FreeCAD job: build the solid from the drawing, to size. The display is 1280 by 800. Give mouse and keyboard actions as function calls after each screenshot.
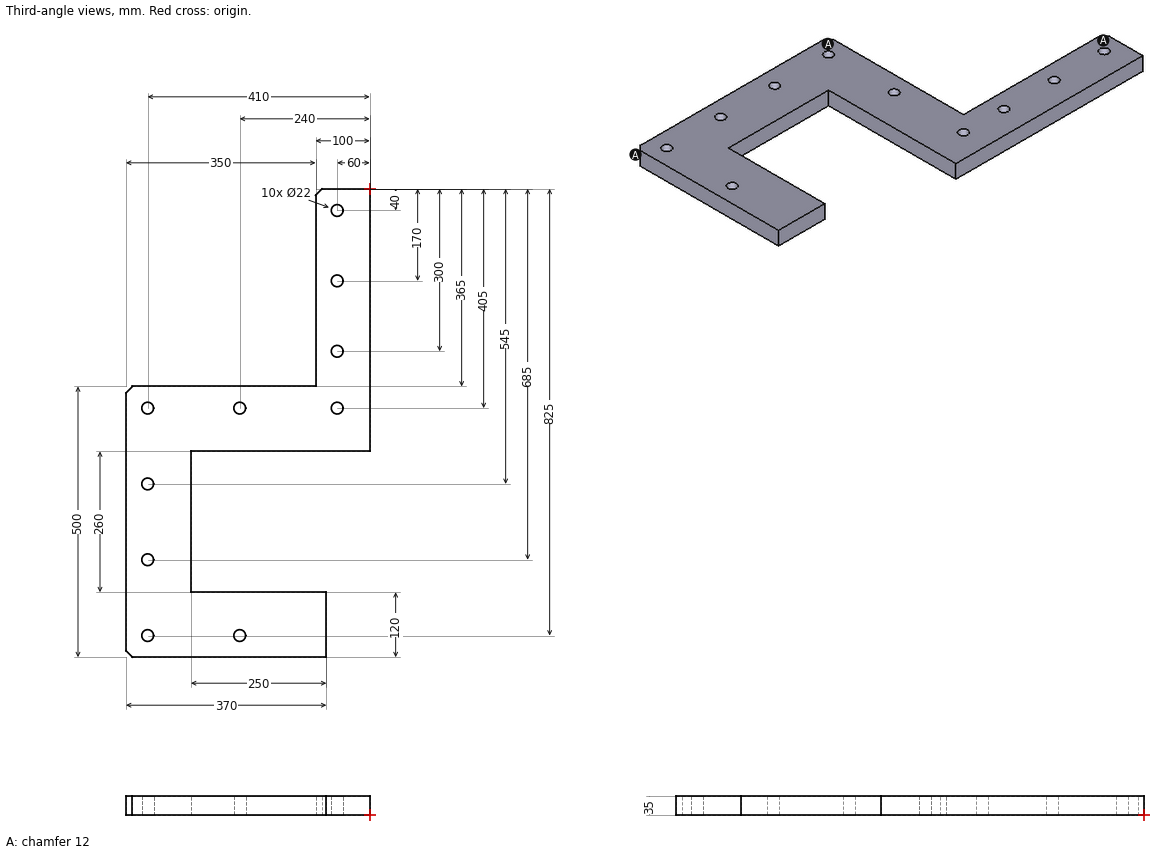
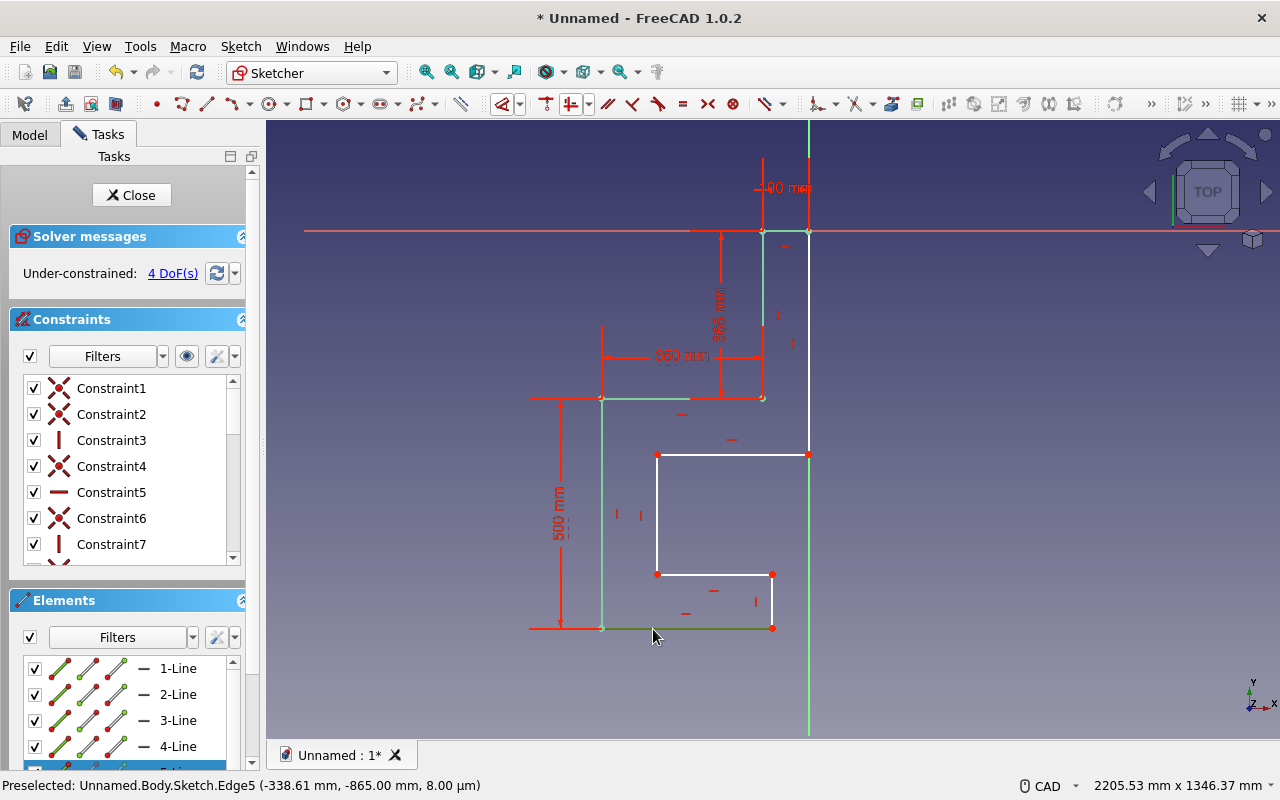
click(520, 104)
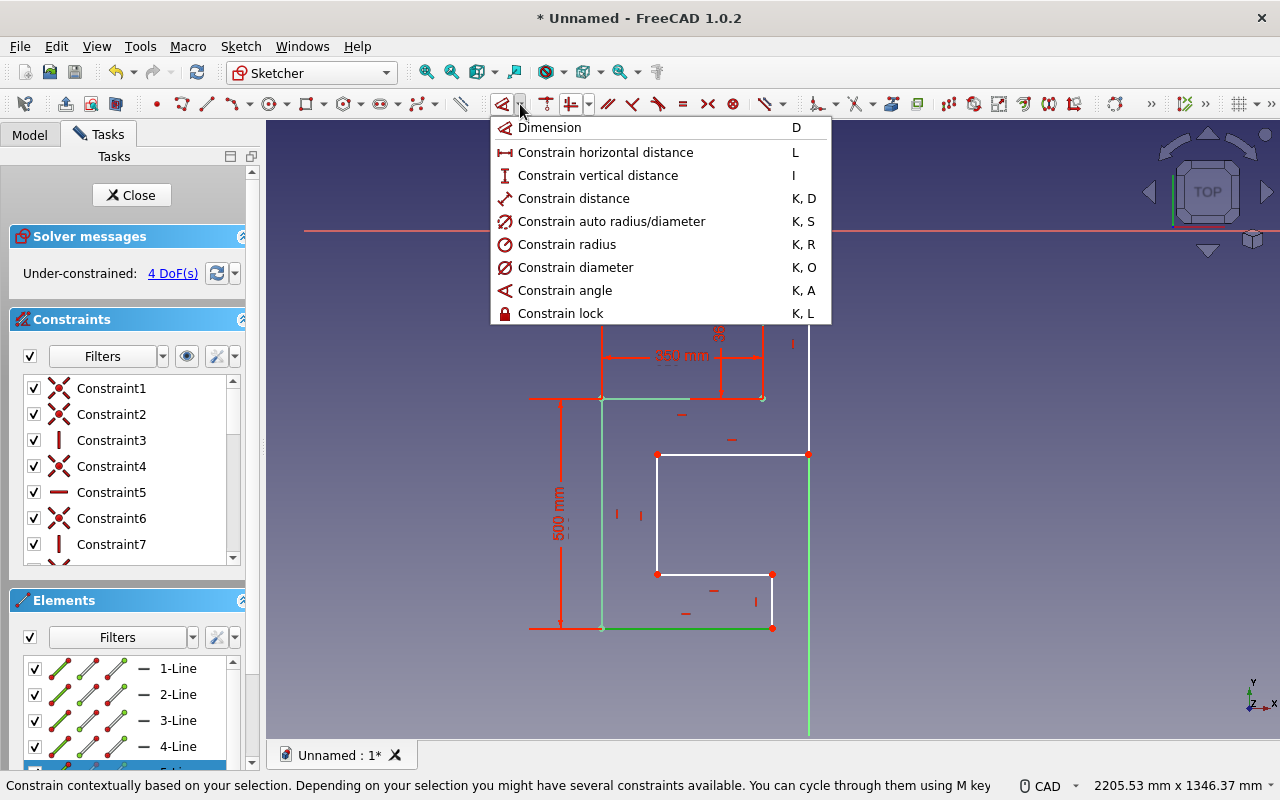
click(661, 152)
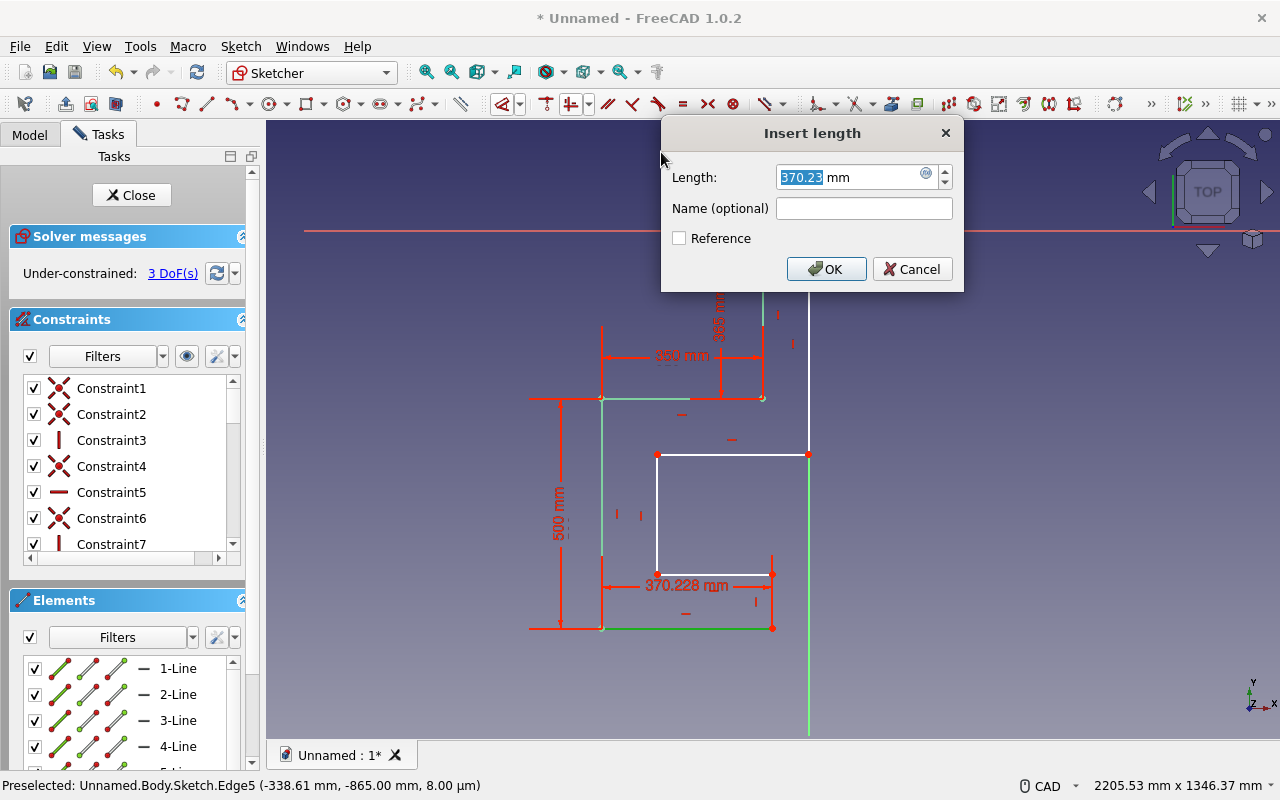
text(370)
key(Return)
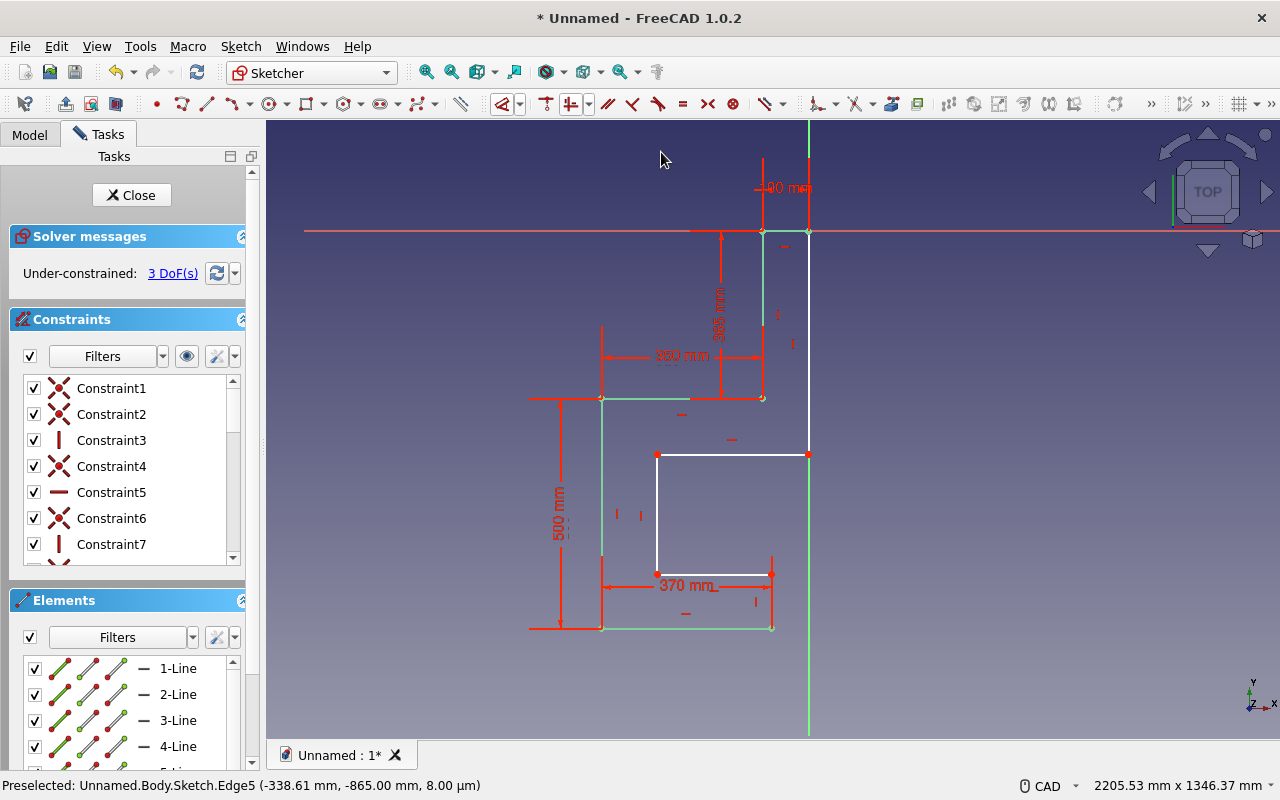
click(772, 613)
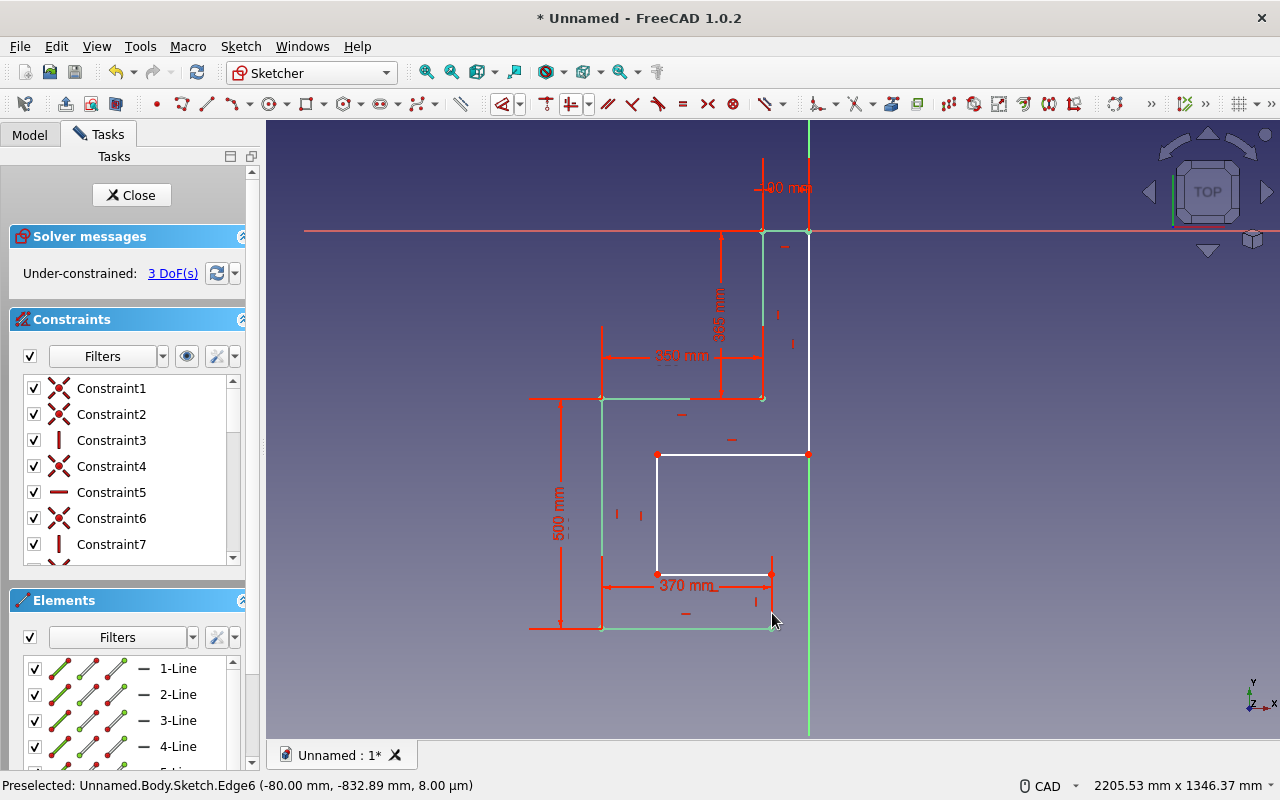
click(520, 104)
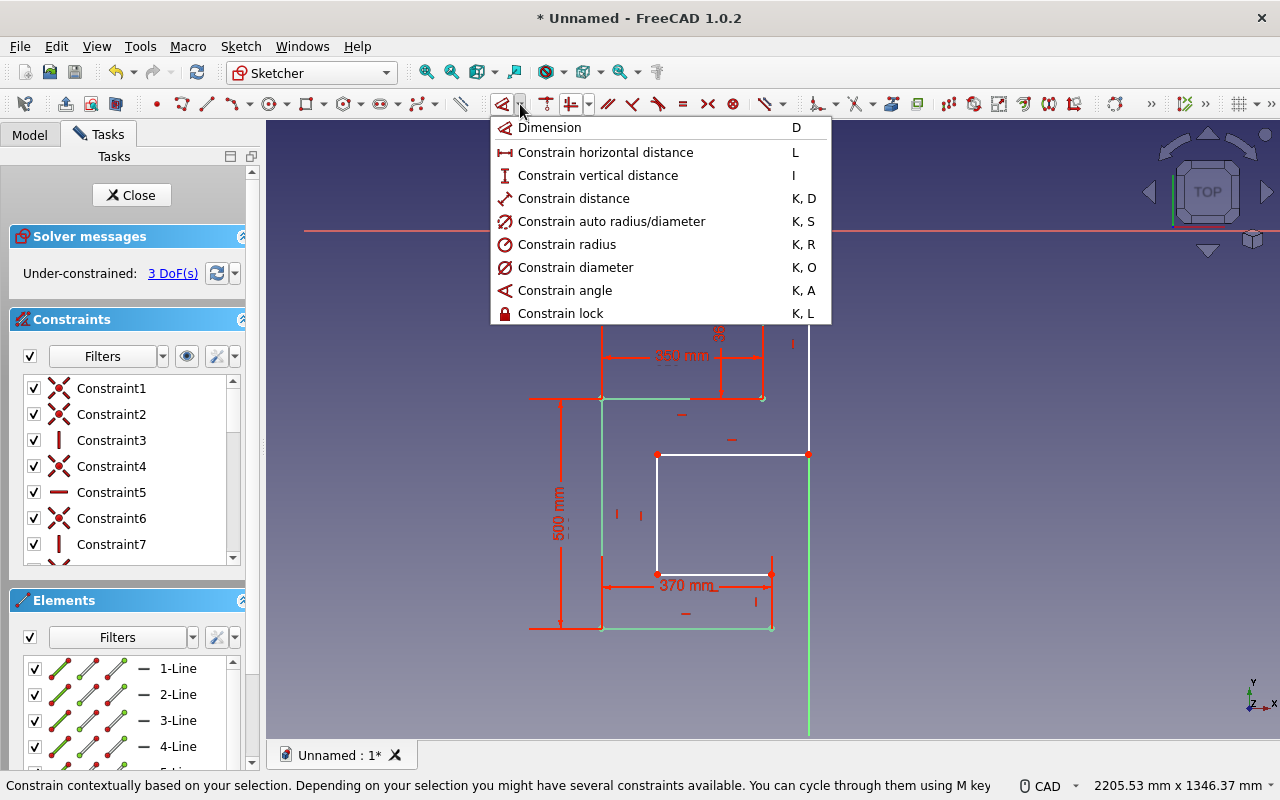
click(661, 176)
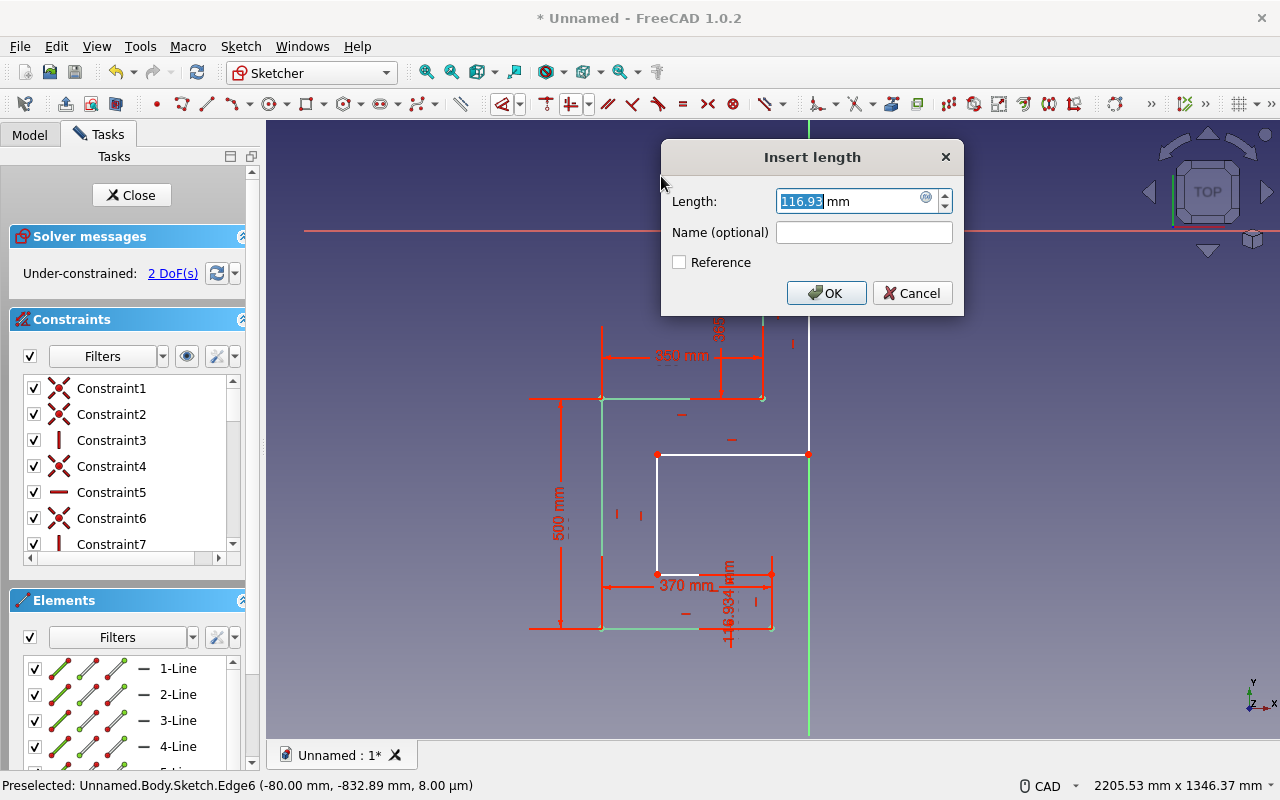
text(120)
key(Return)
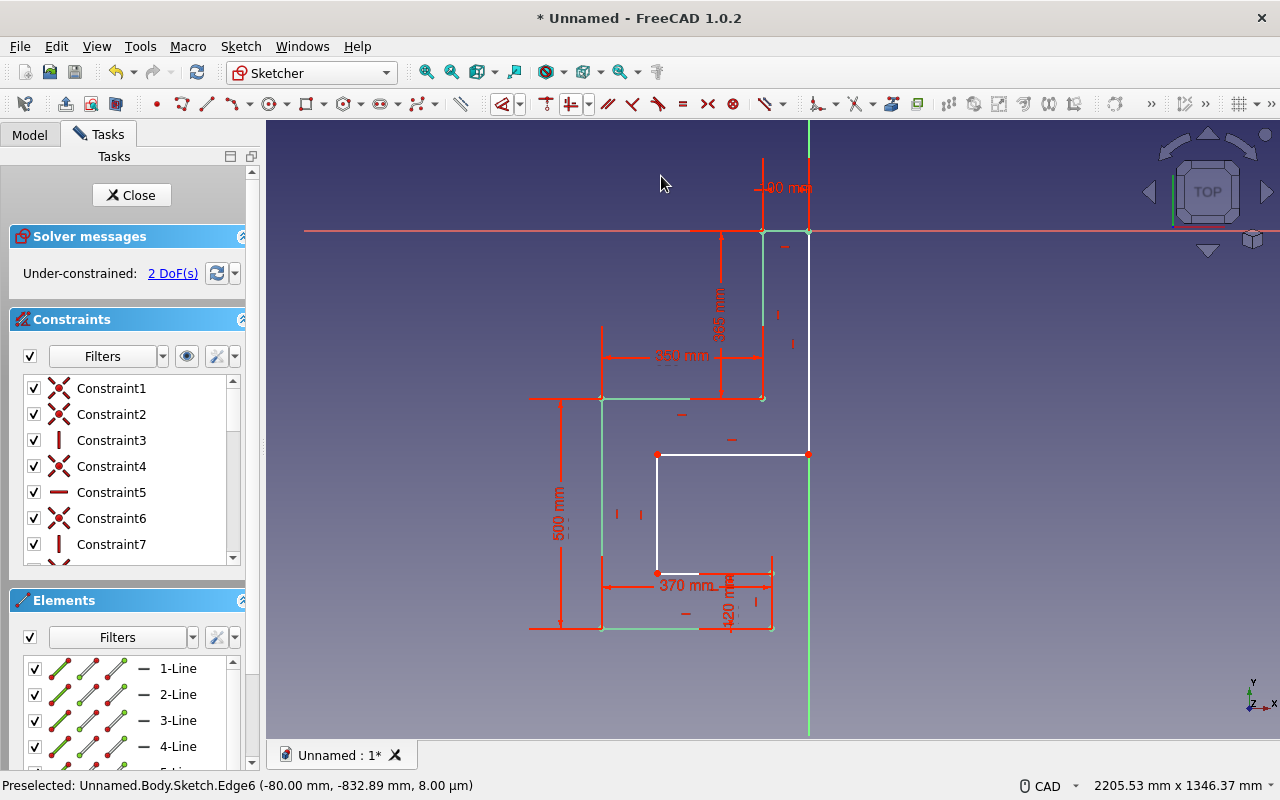
click(691, 574)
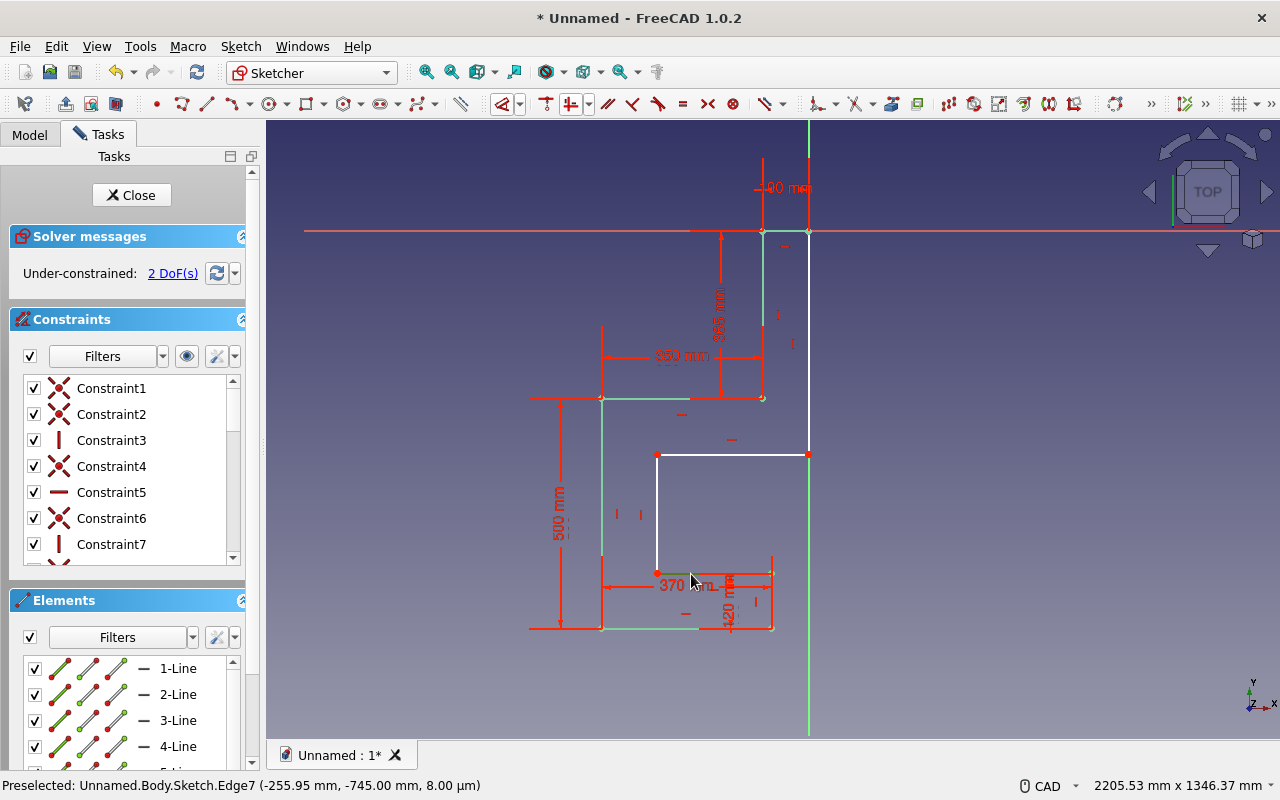
click(520, 104)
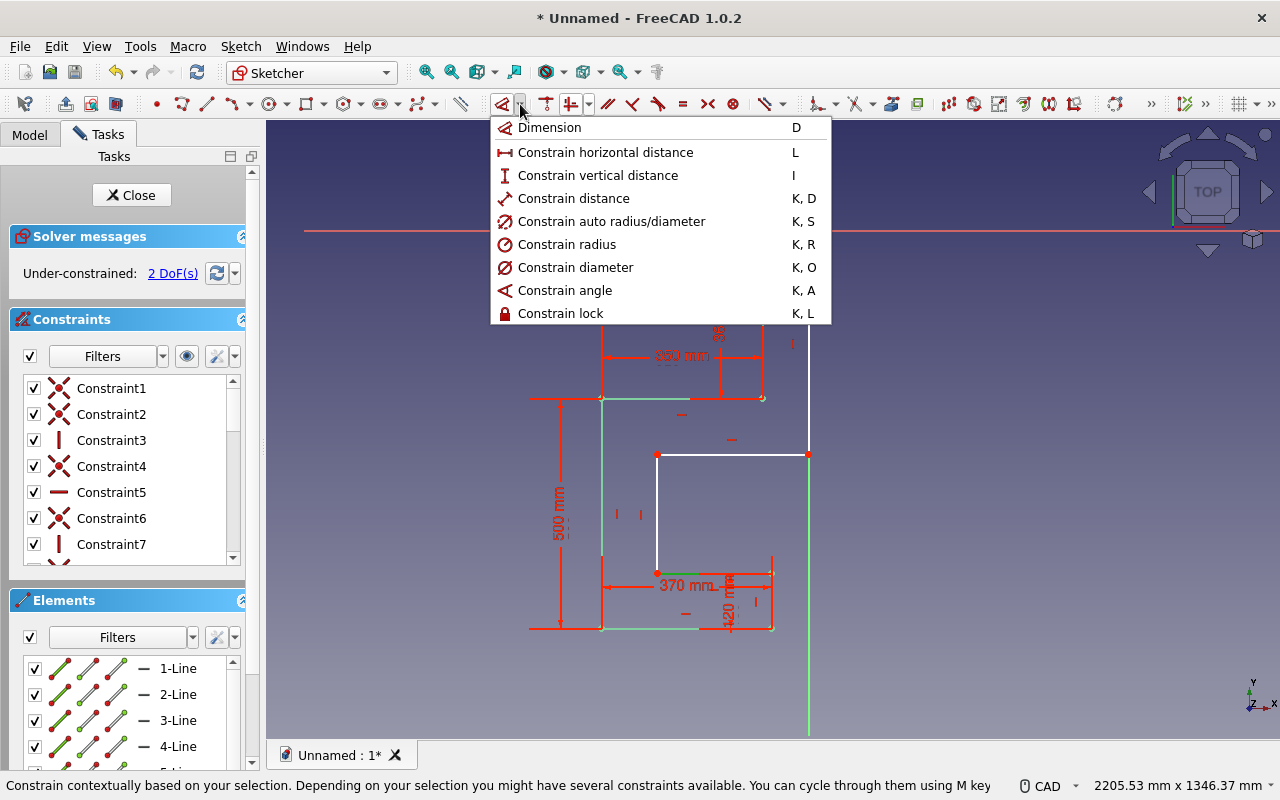
click(661, 152)